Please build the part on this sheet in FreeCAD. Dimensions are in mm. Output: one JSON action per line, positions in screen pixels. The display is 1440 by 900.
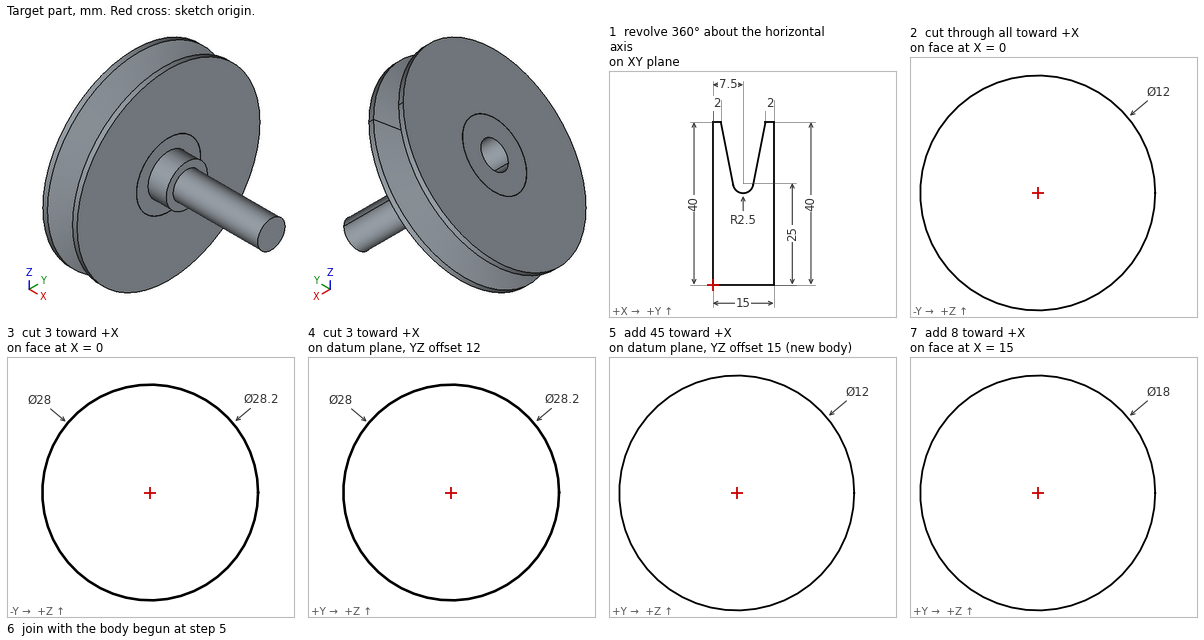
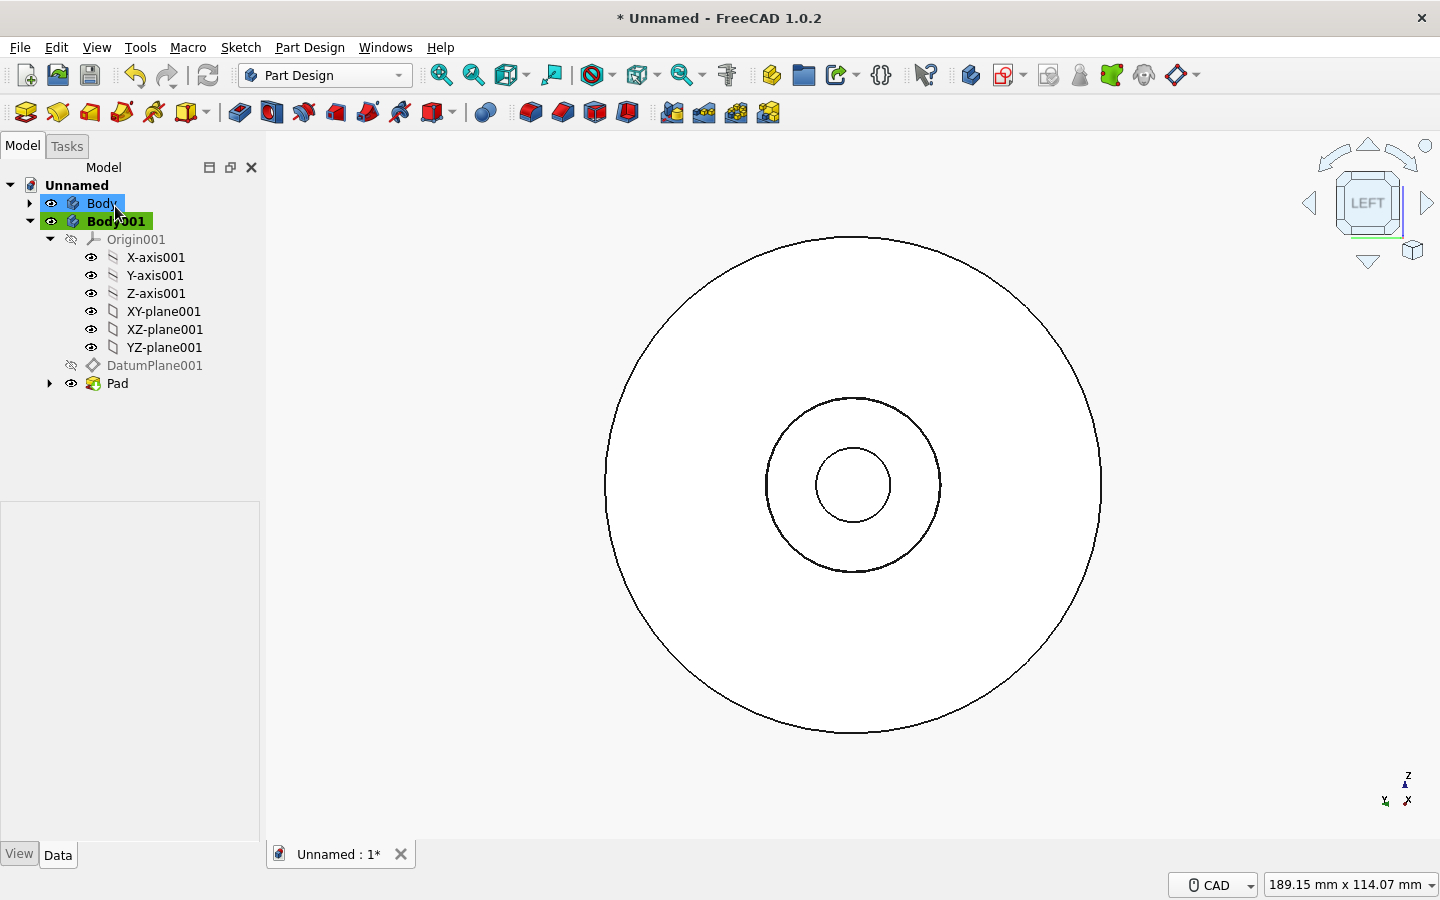
{"action": "key", "text": "v f"}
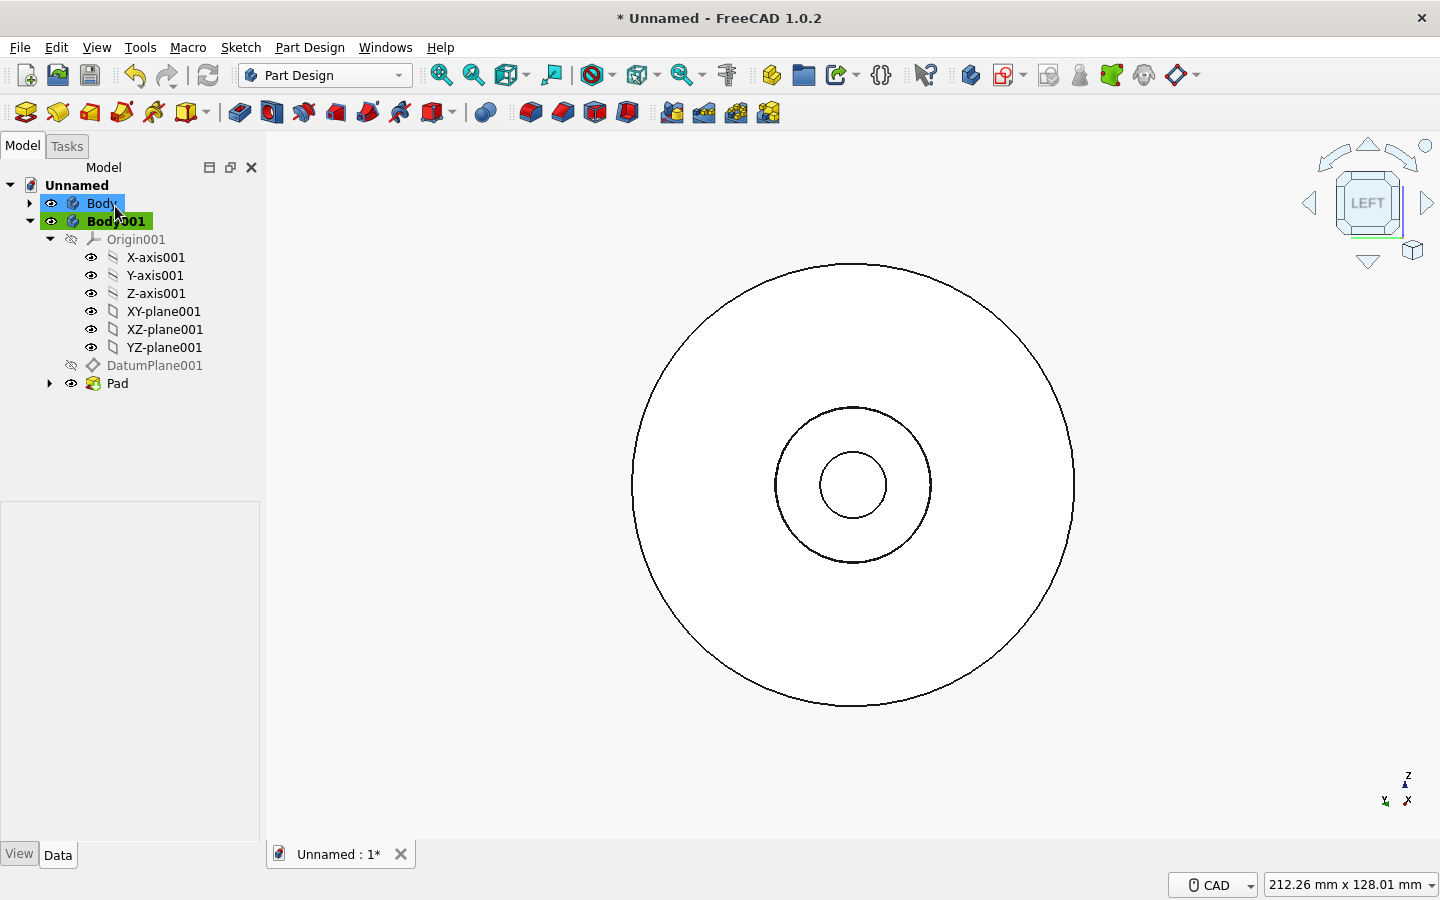
{"action": "double_click", "coordinate": [96, 203]}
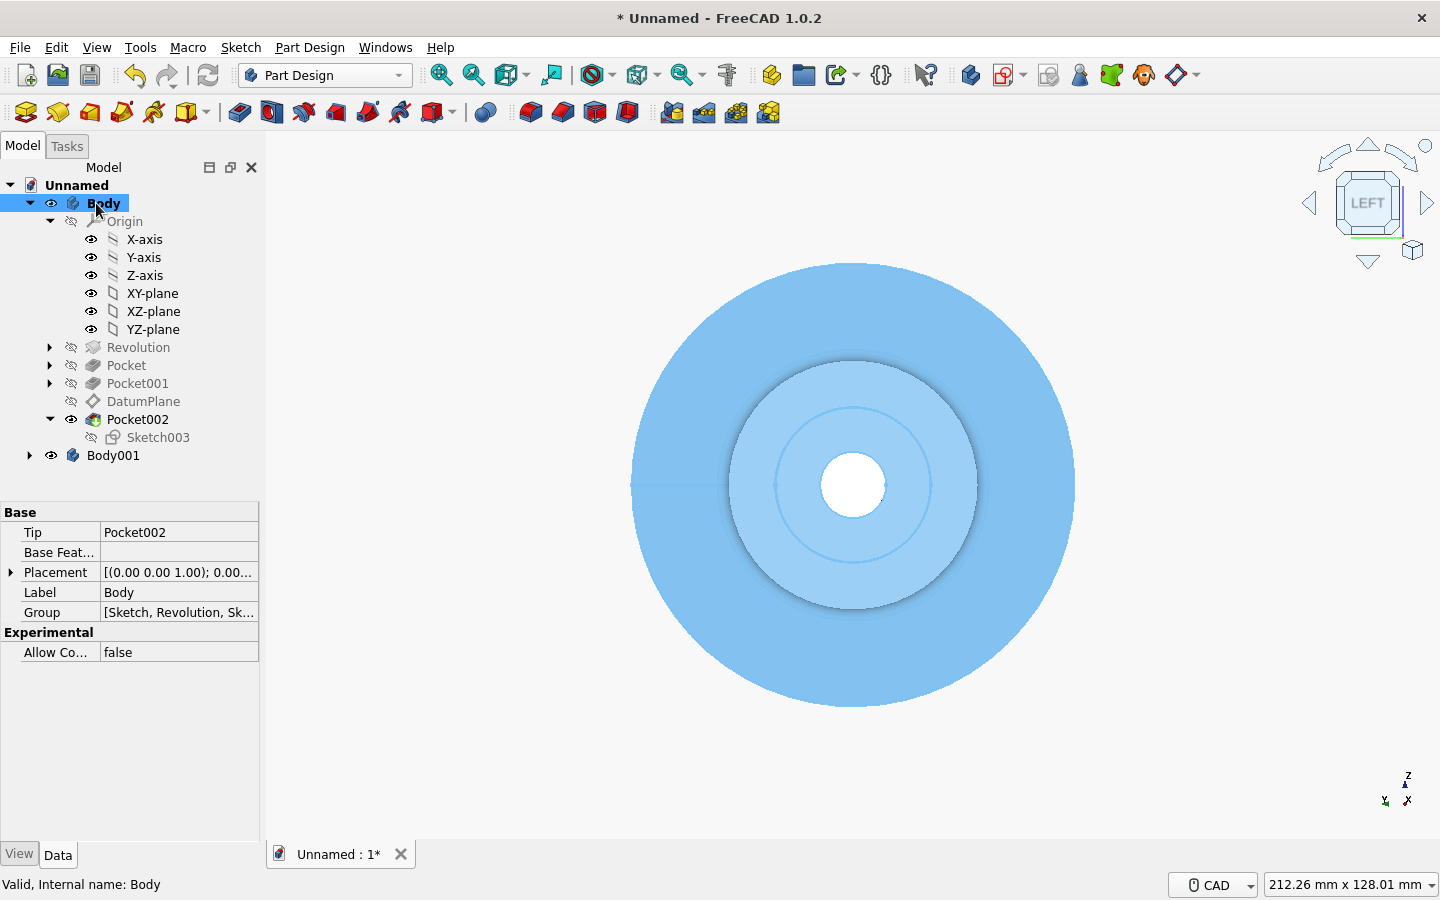
{"action": "left_click", "coordinate": [96, 203]}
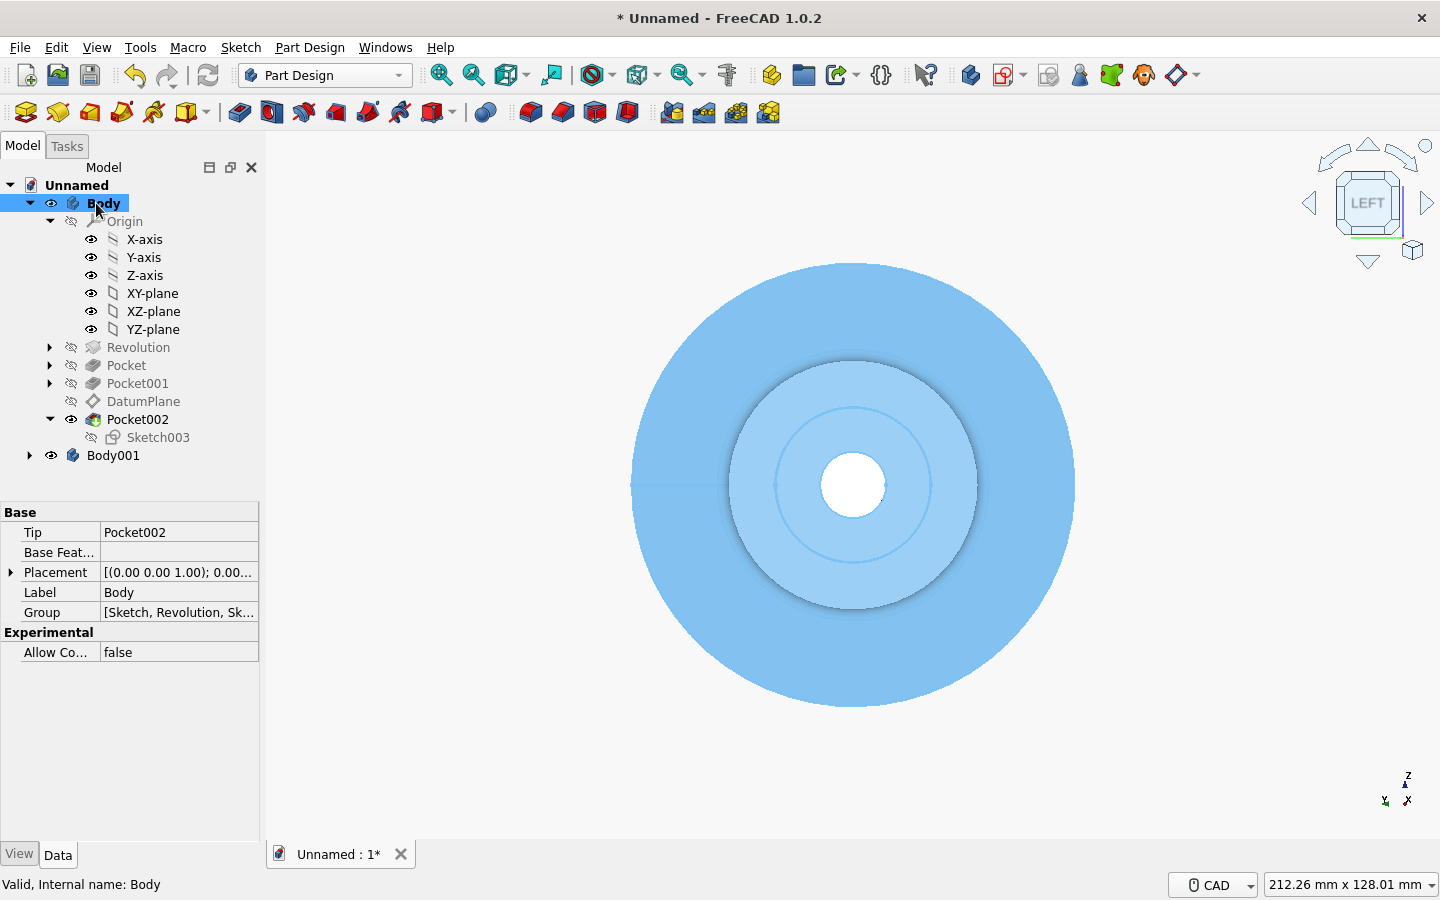
{"action": "left_click", "coordinate": [146, 652]}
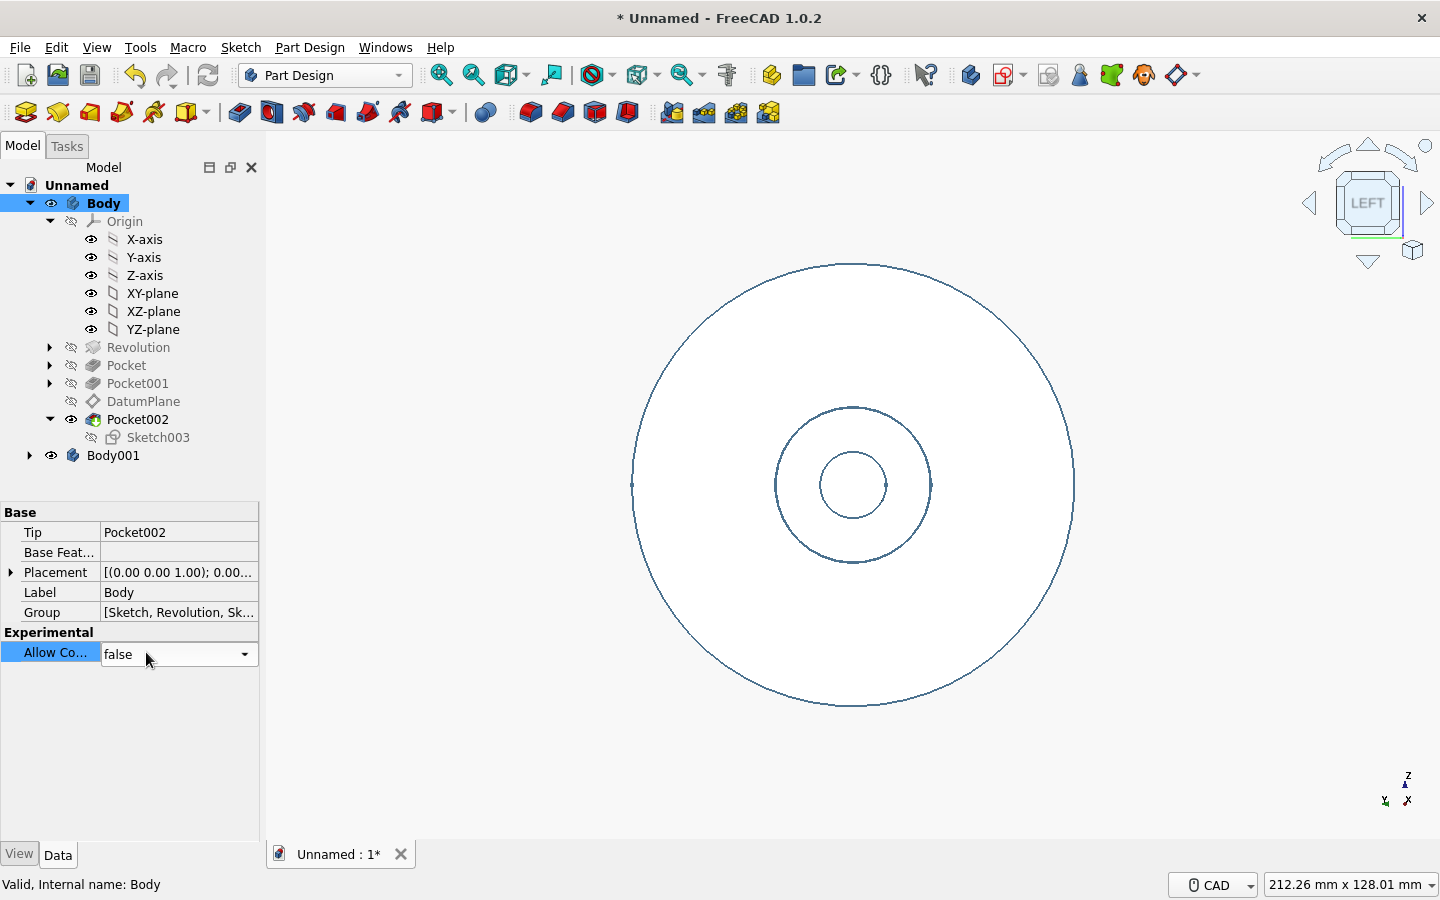
{"action": "left_click", "coordinate": [146, 652]}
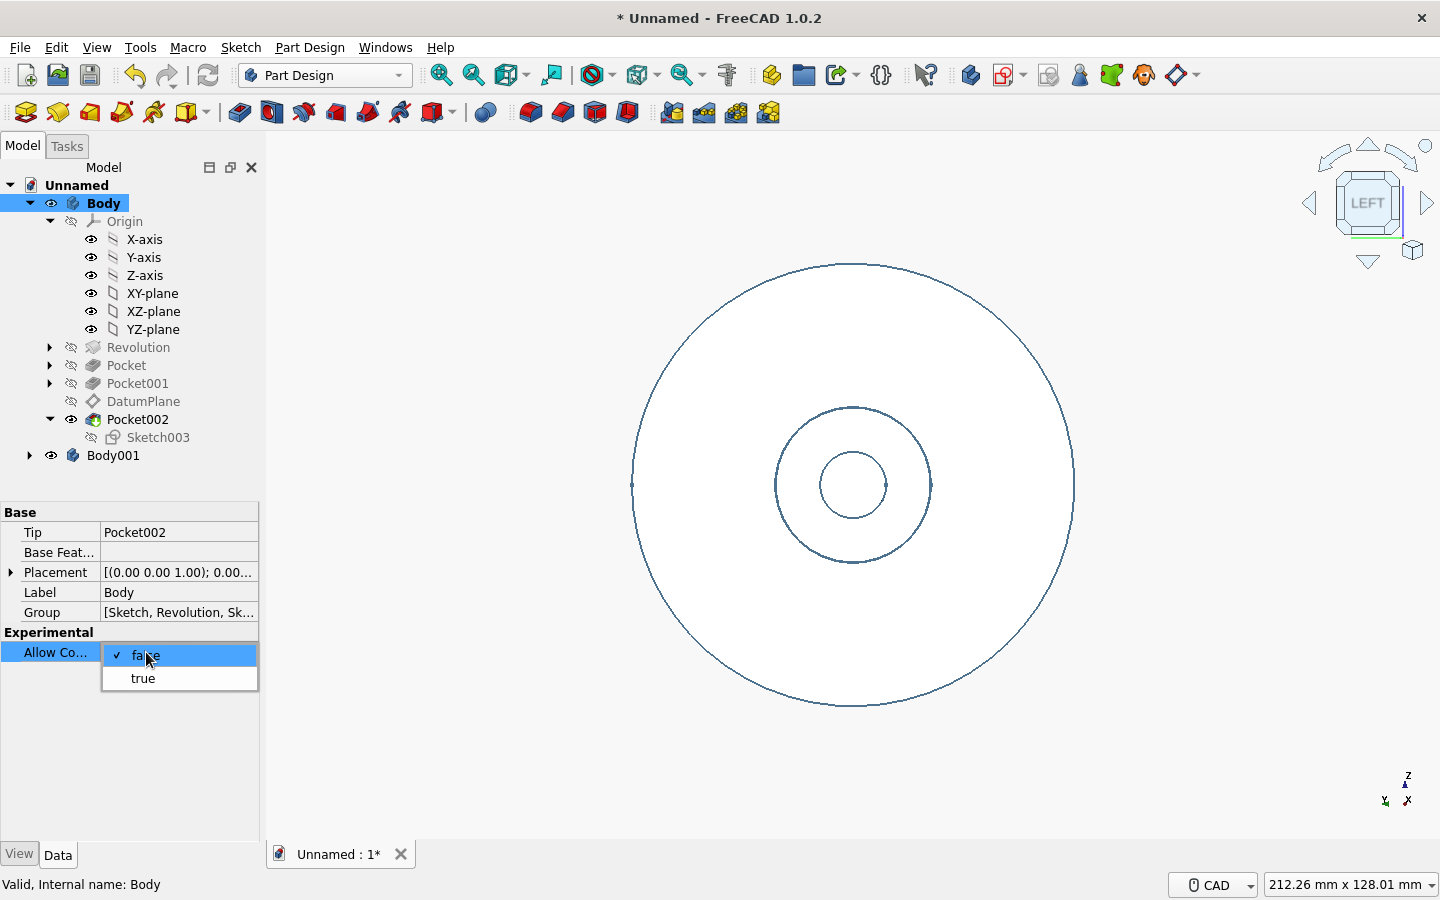
{"action": "left_click", "coordinate": [179, 678]}
{"action": "key", "text": "Return"}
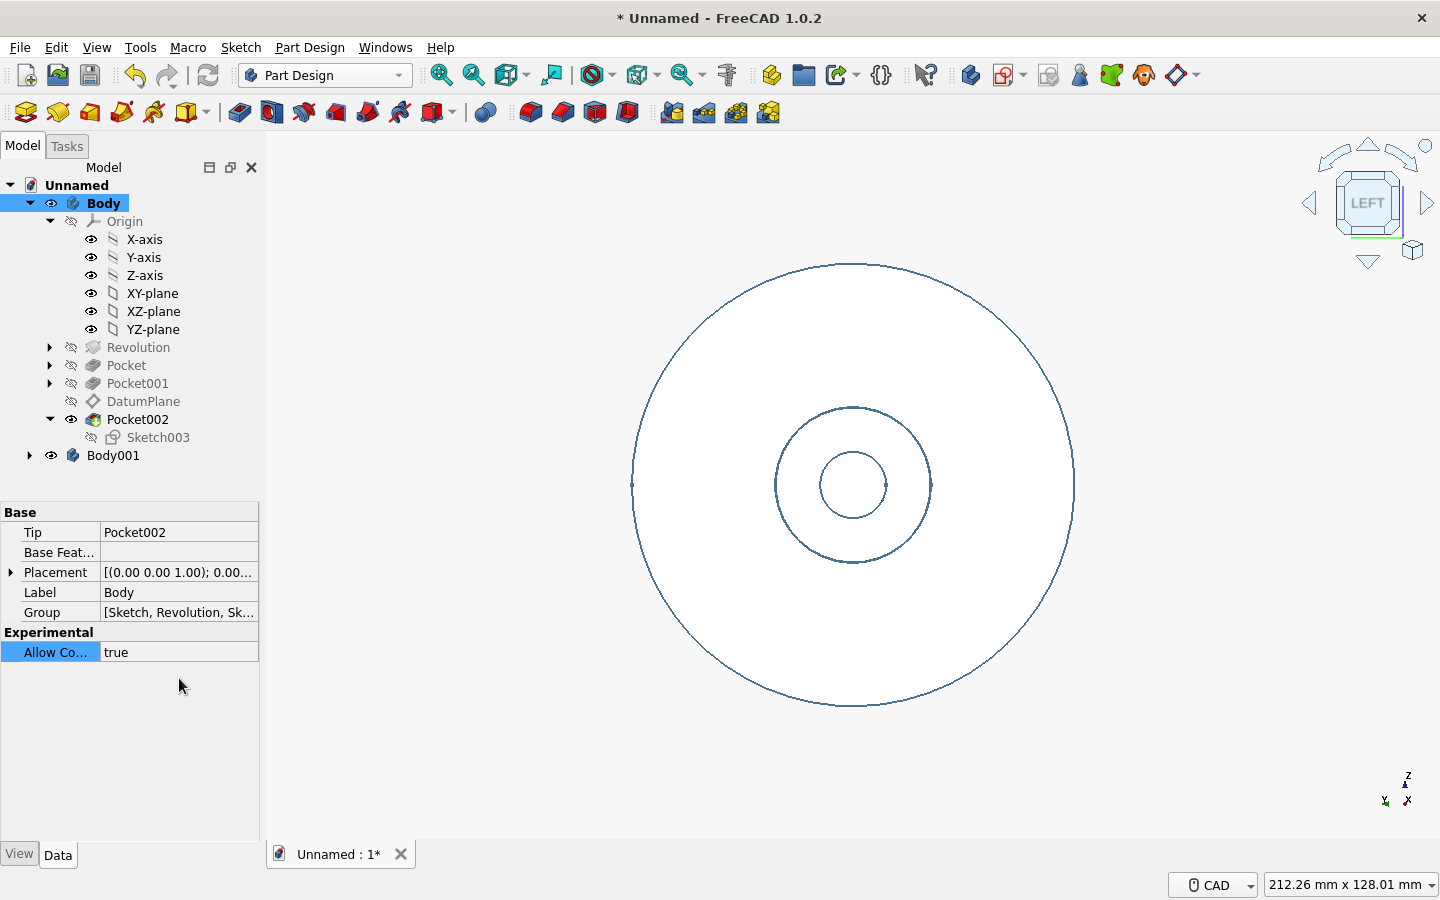
{"action": "left_click", "coordinate": [96, 455]}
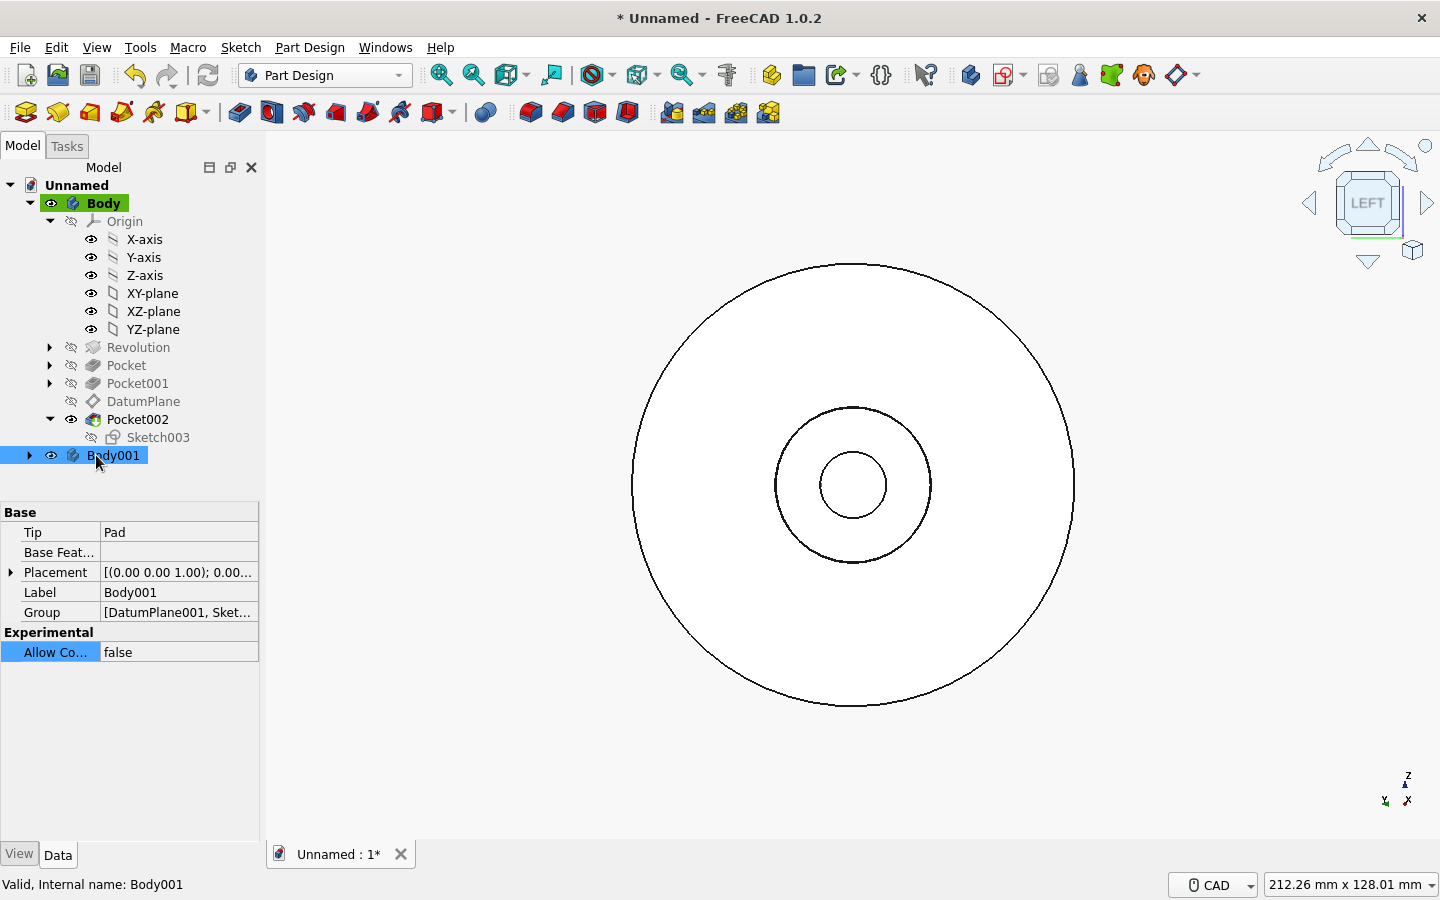
{"action": "left_click", "coordinate": [486, 112]}